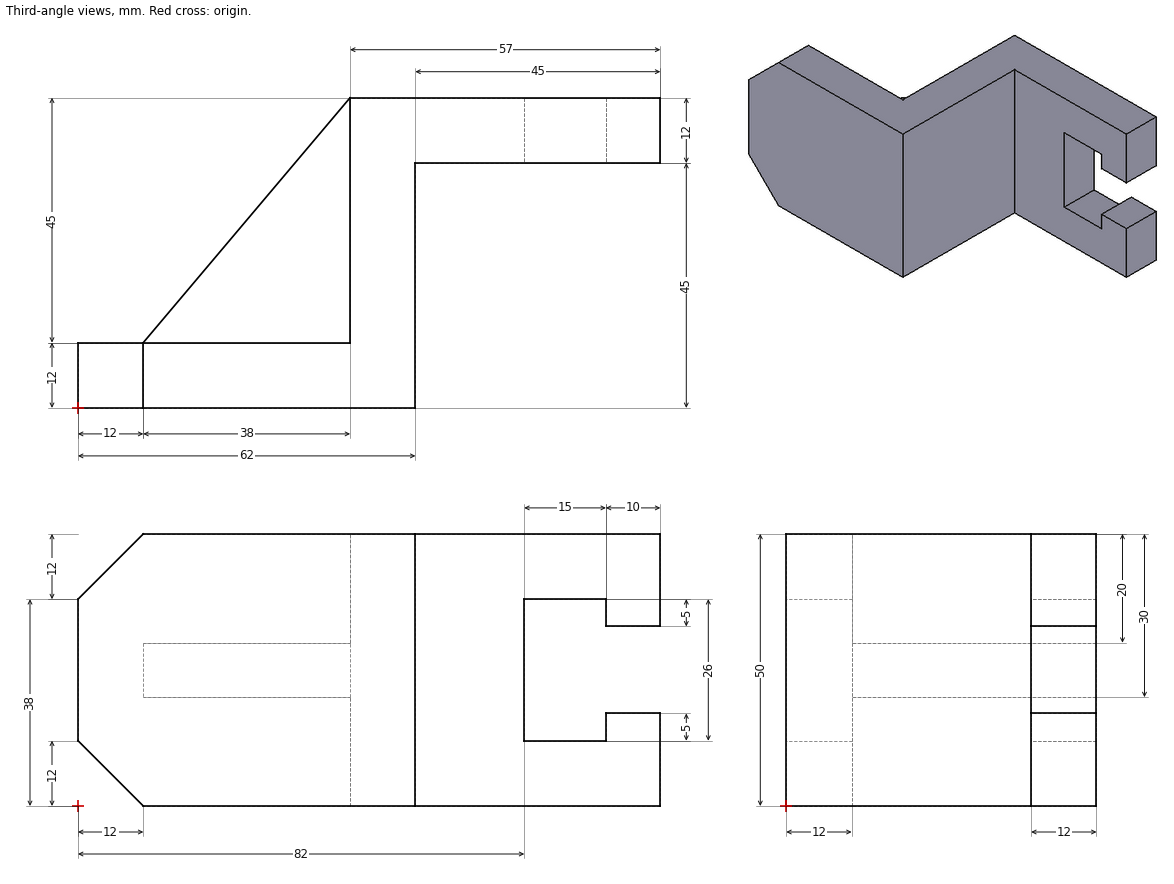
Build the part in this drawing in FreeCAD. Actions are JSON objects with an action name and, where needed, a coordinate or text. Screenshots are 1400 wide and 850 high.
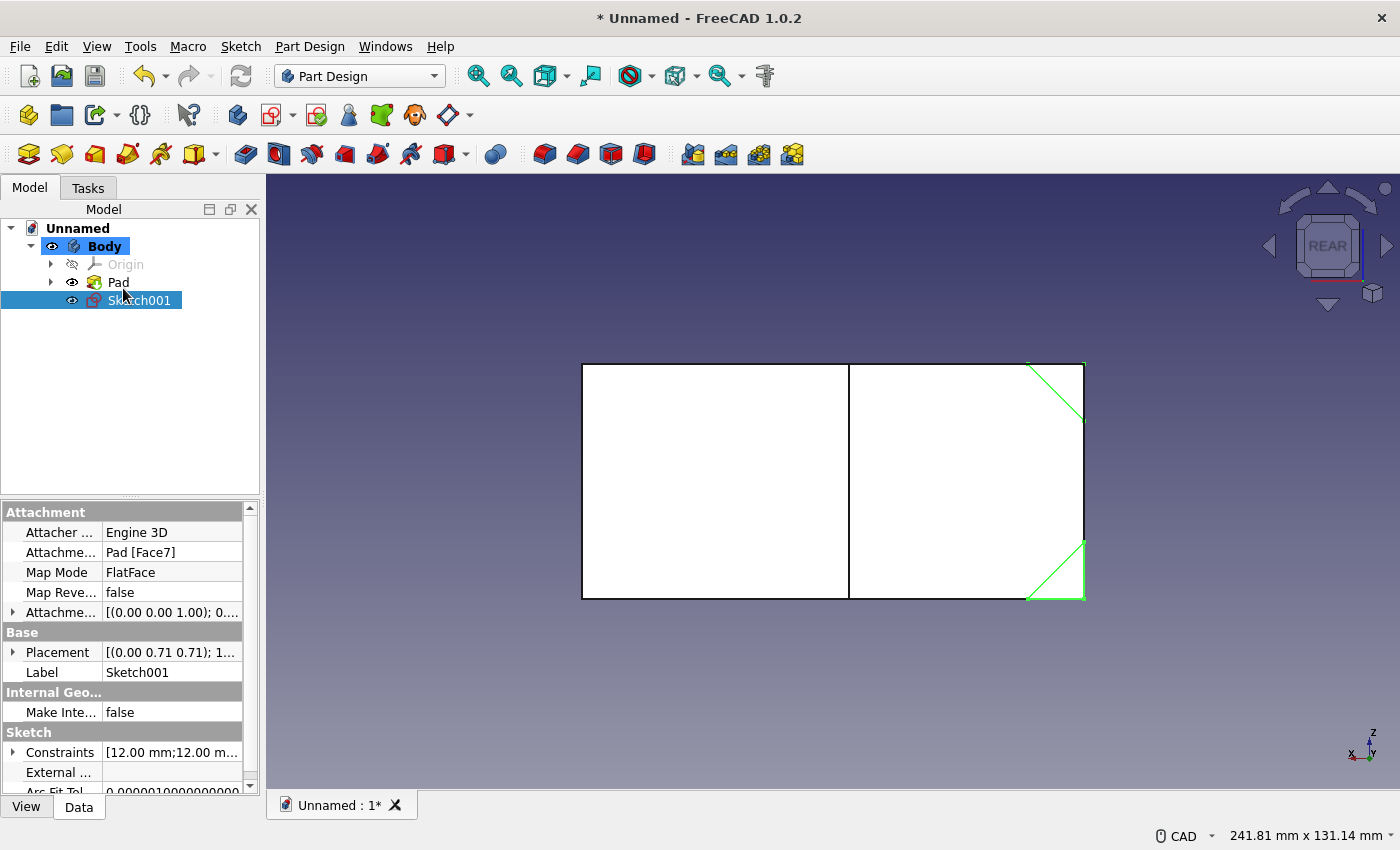
{"action": "left_click", "coordinate": [246, 154]}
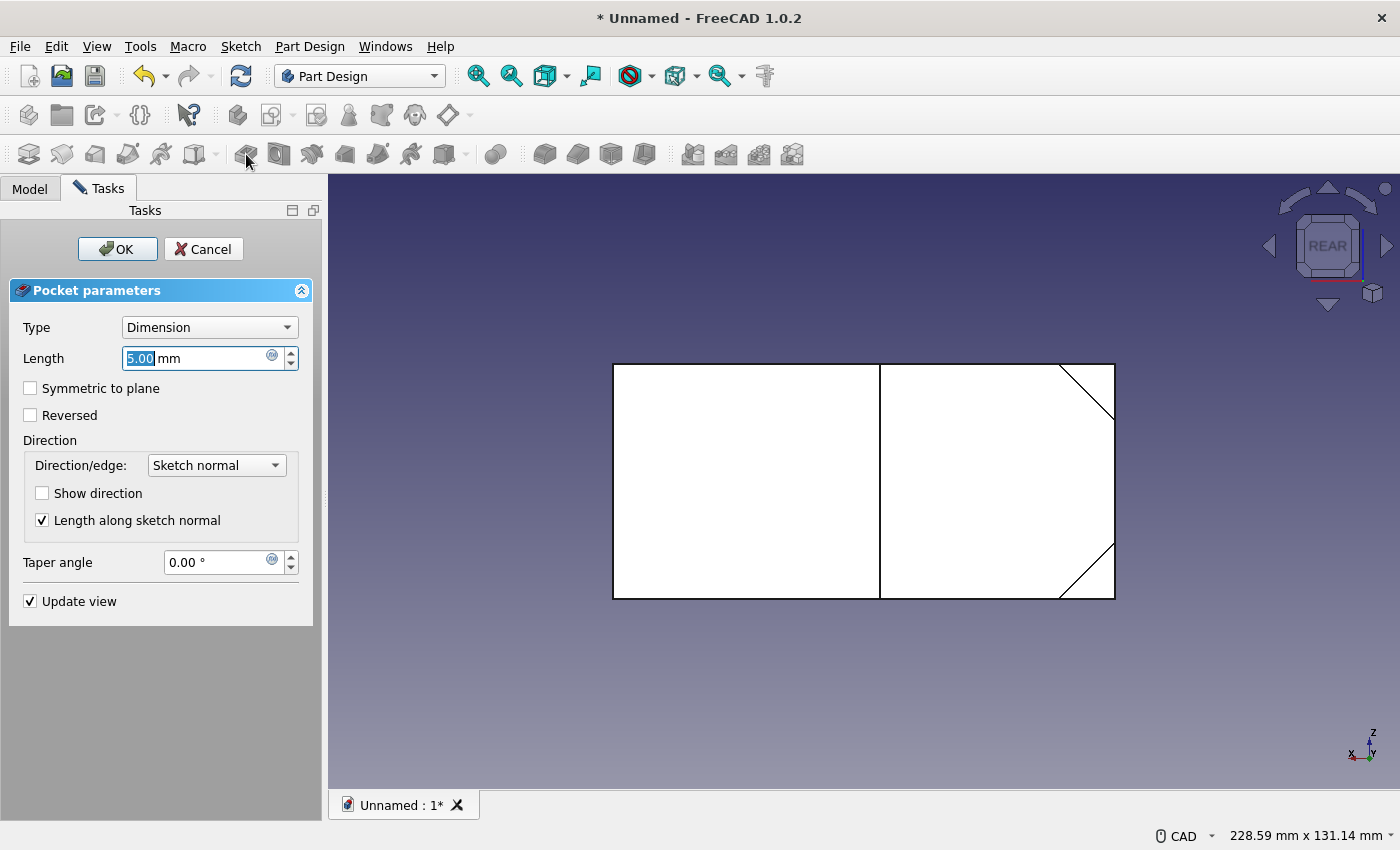
{"action": "type", "text": "12"}
{"action": "key", "text": "Tab"}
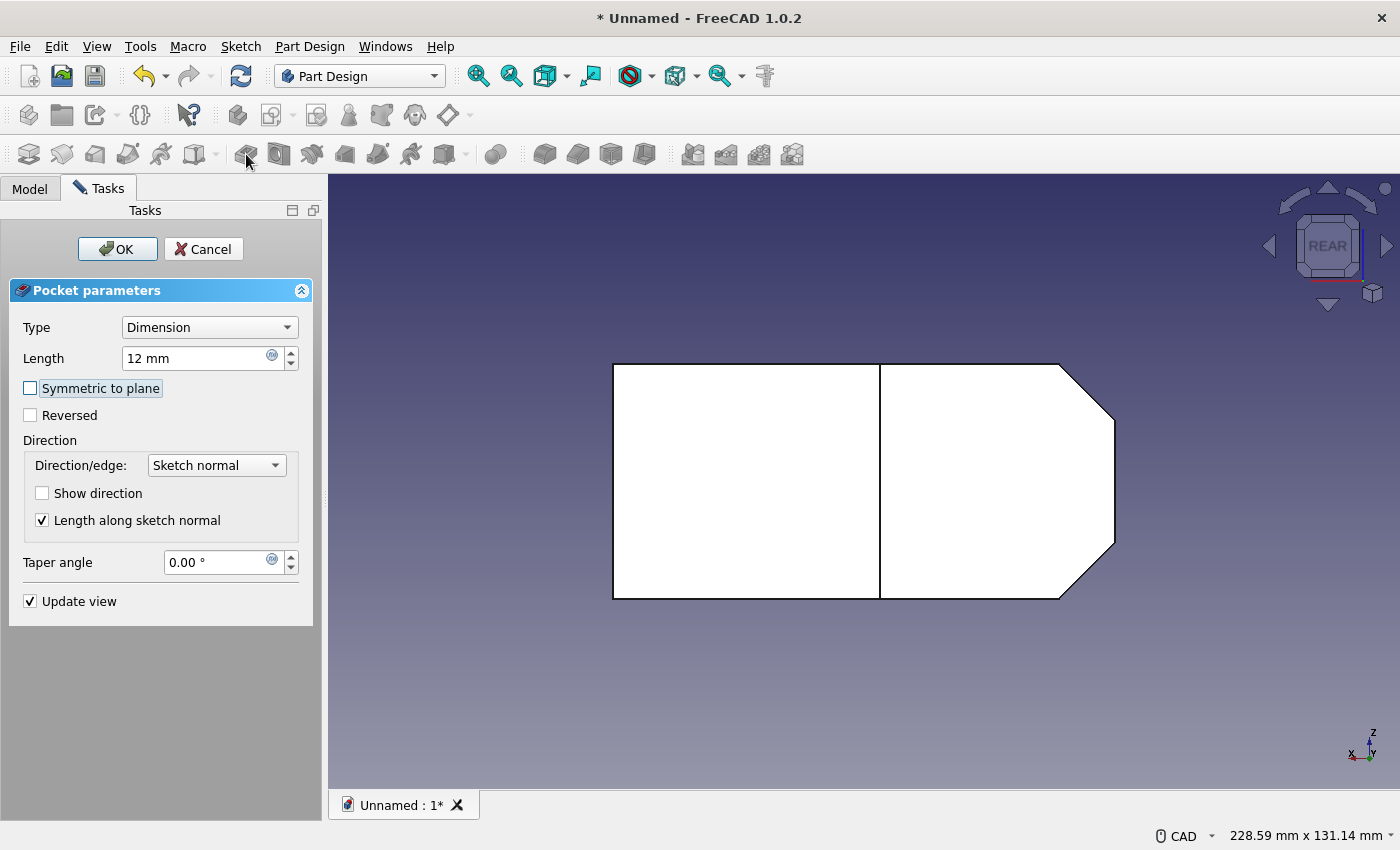
{"action": "left_click", "coordinate": [118, 249]}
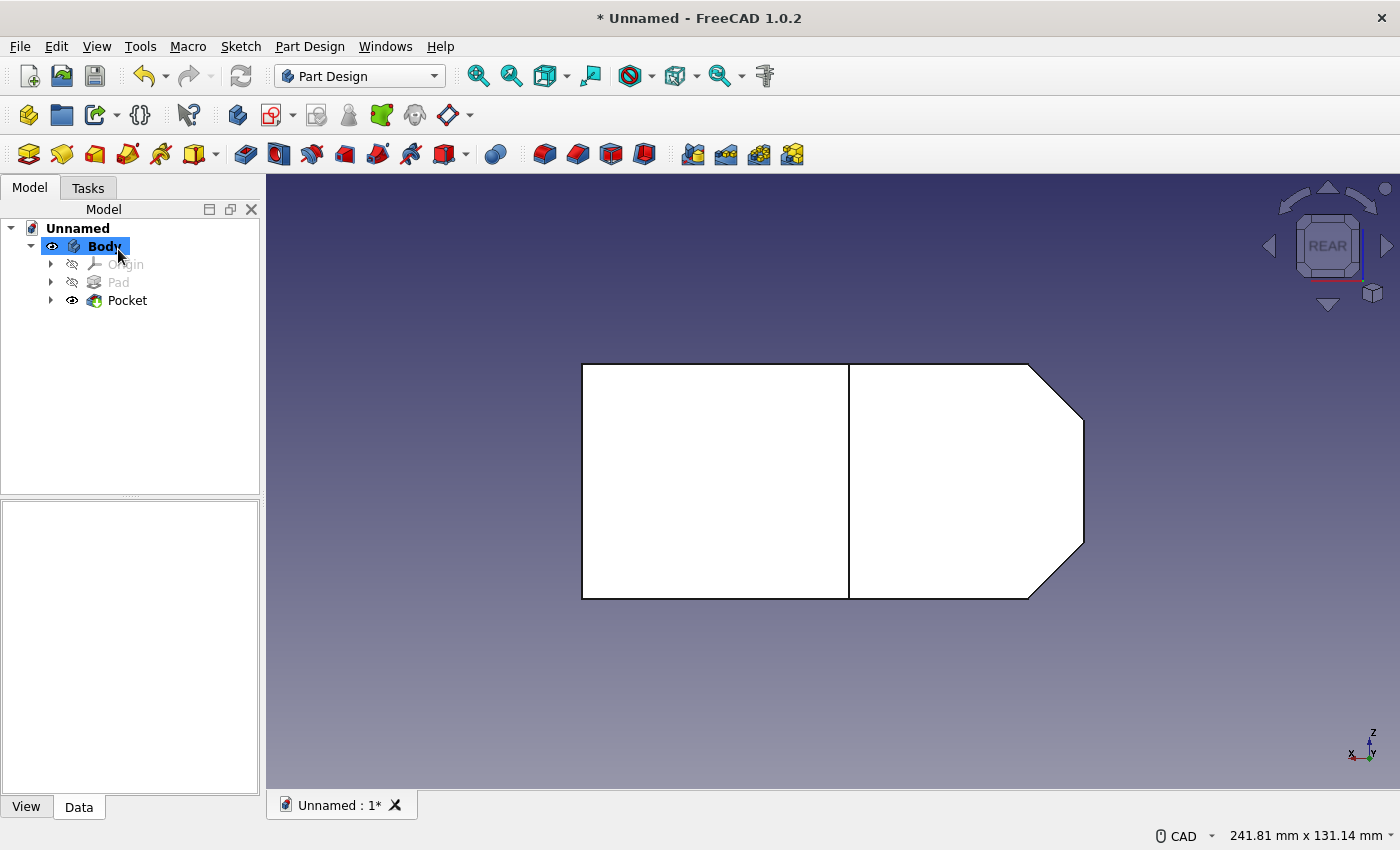
{"action": "left_click", "coordinate": [479, 76]}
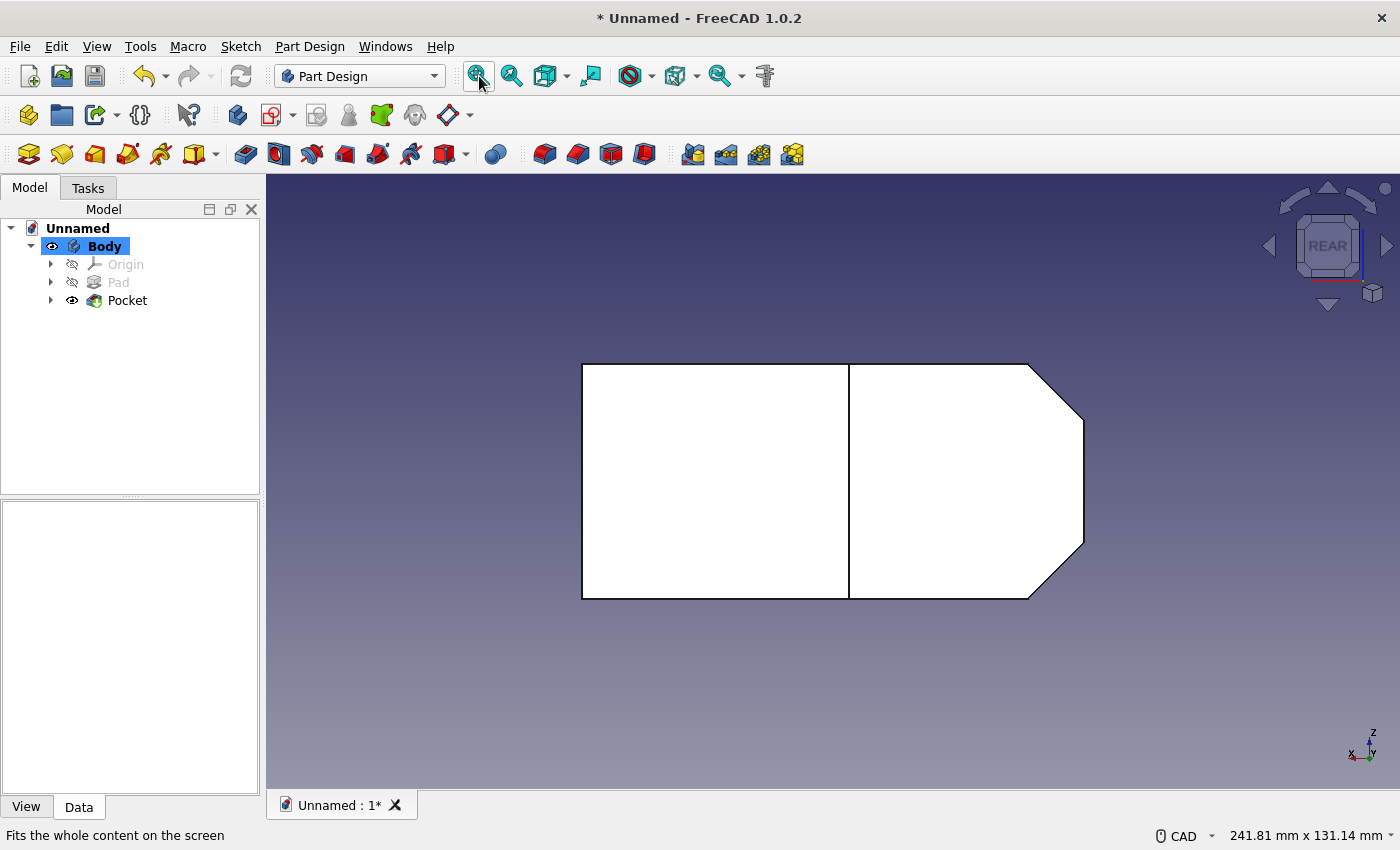
{"action": "left_click", "coordinate": [716, 480]}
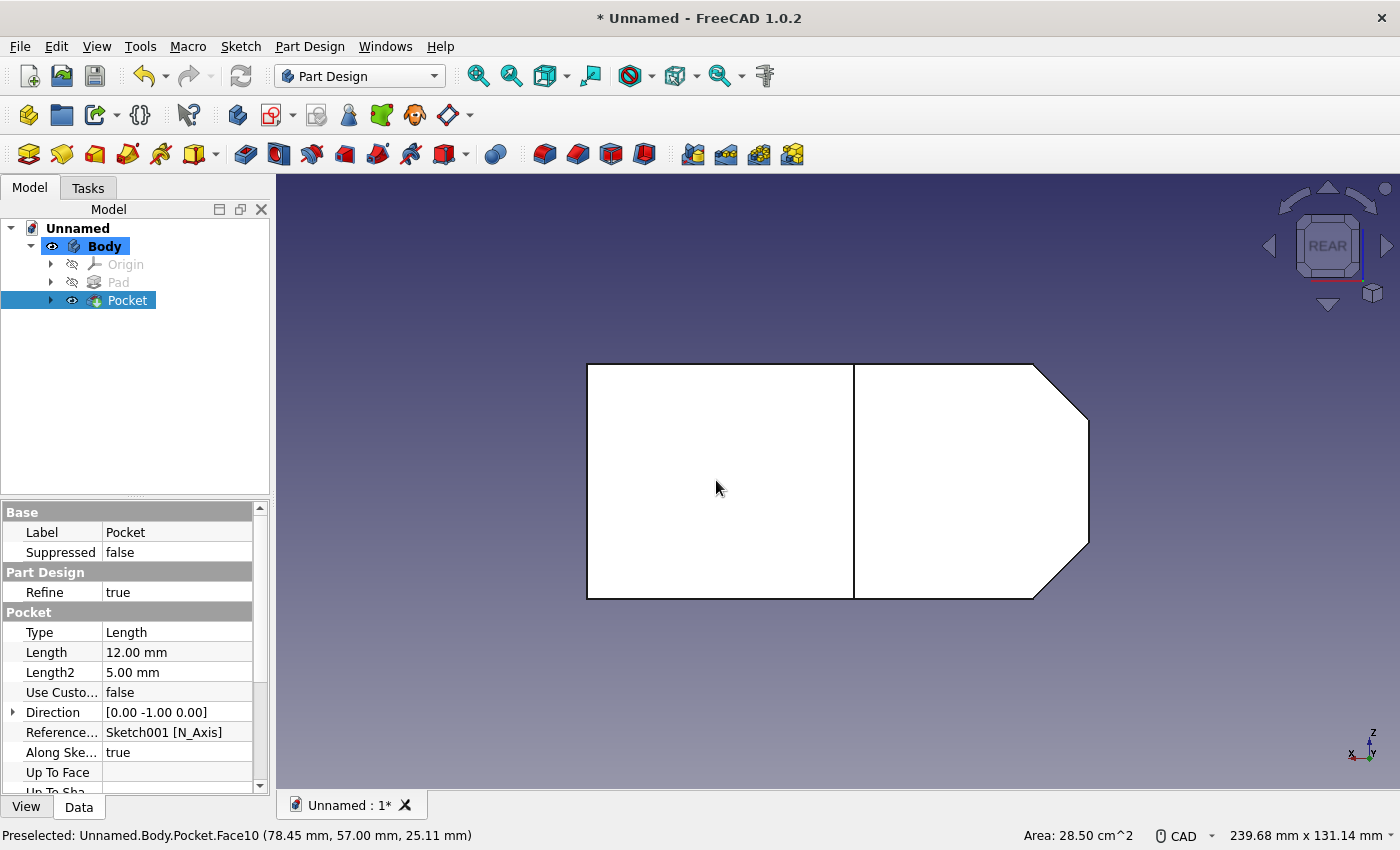
{"action": "left_click", "coordinate": [270, 116]}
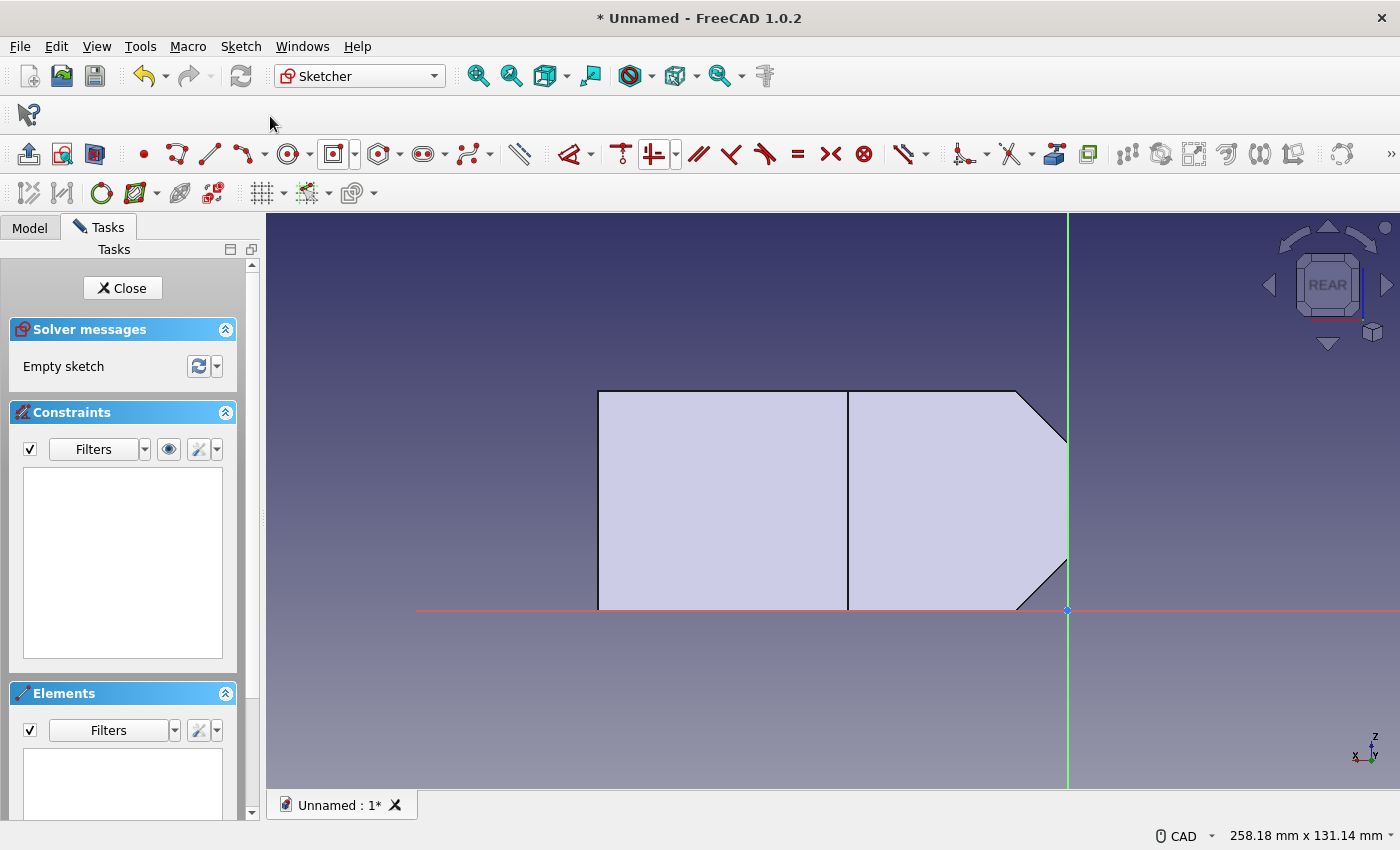
{"action": "scroll", "coordinate": [605, 501], "scroll_direction": "up", "scroll_amount": 6}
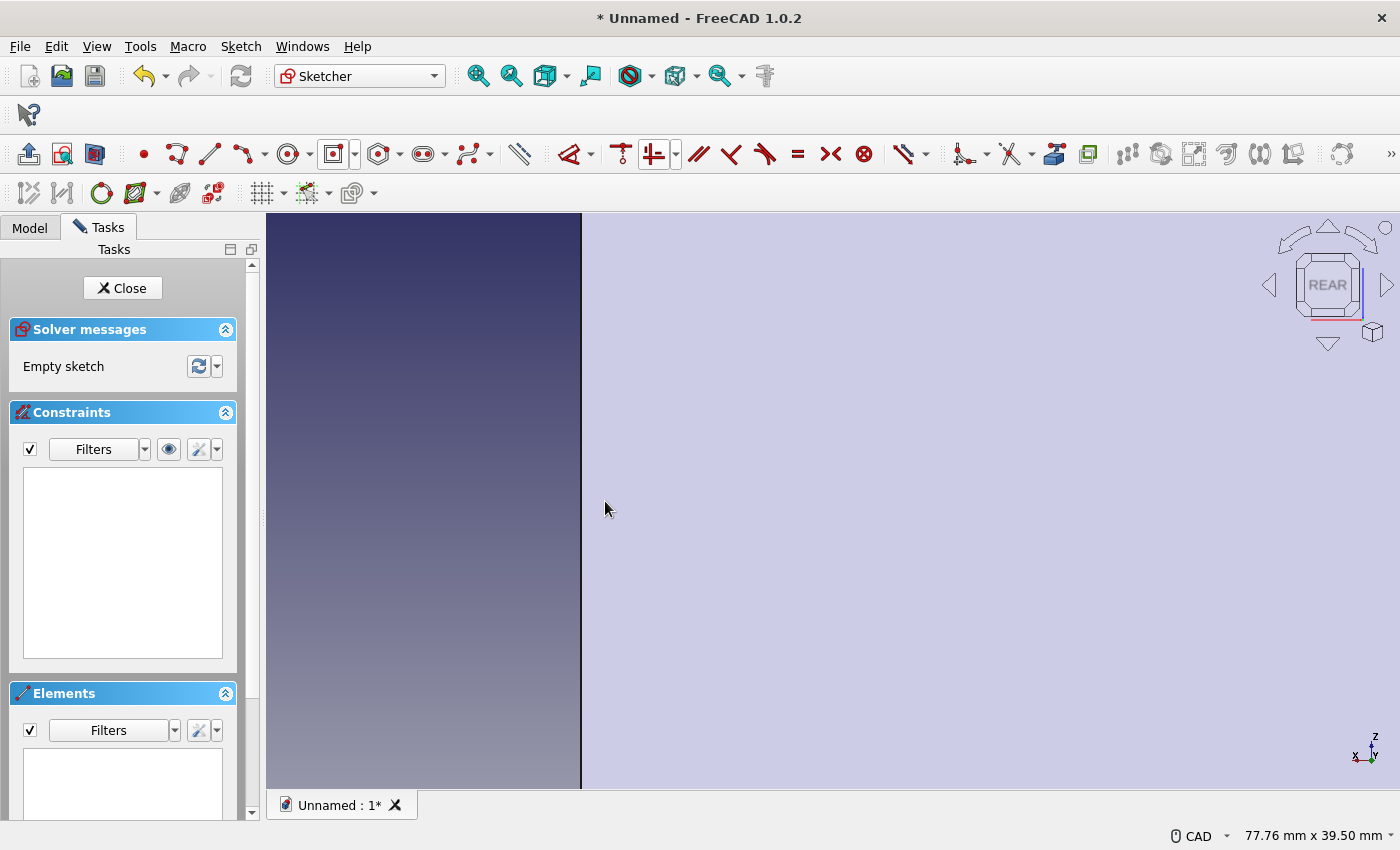
{"action": "left_click", "coordinate": [177, 154]}